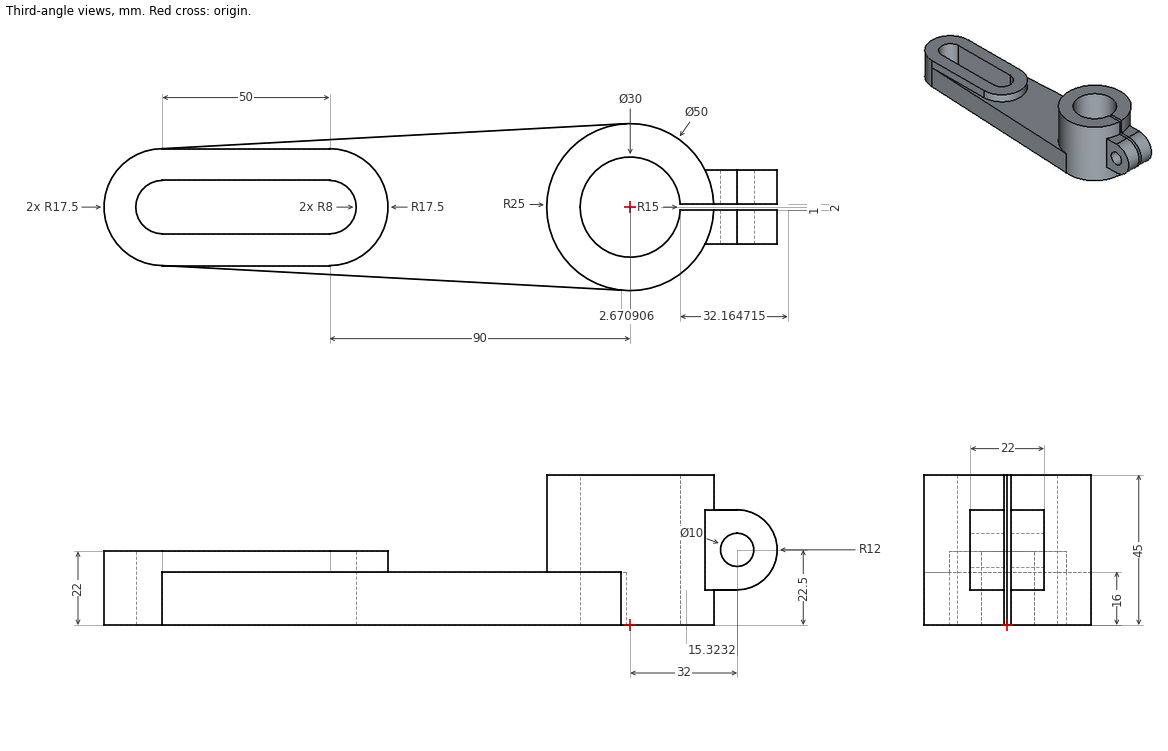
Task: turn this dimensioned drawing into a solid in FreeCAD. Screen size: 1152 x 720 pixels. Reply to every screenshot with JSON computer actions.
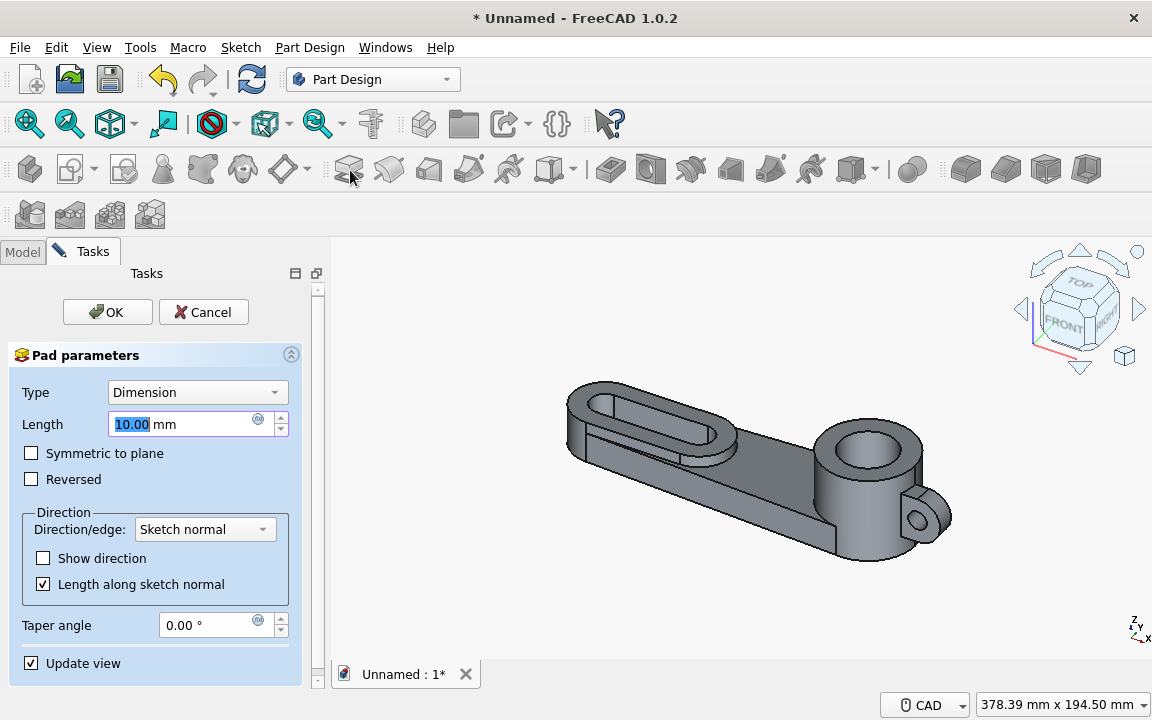
{"action": "type", "text": "22"}
{"action": "key", "text": "Tab"}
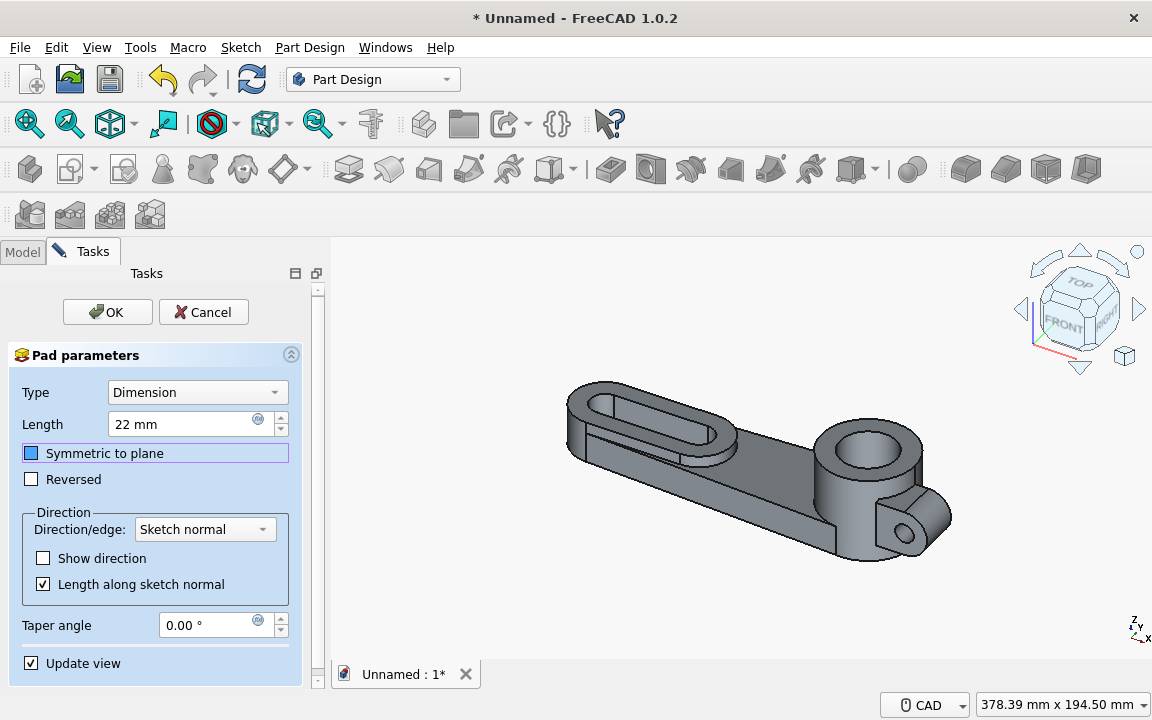
{"action": "left_click", "coordinate": [30, 453]}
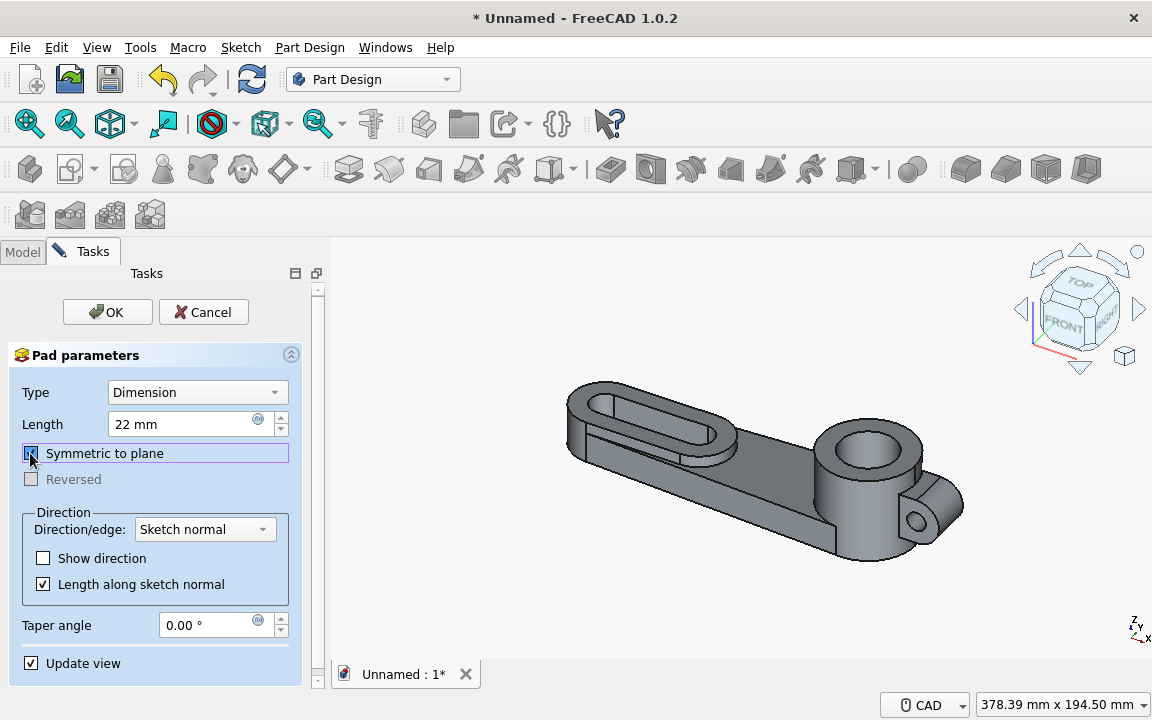
{"action": "left_click", "coordinate": [108, 312]}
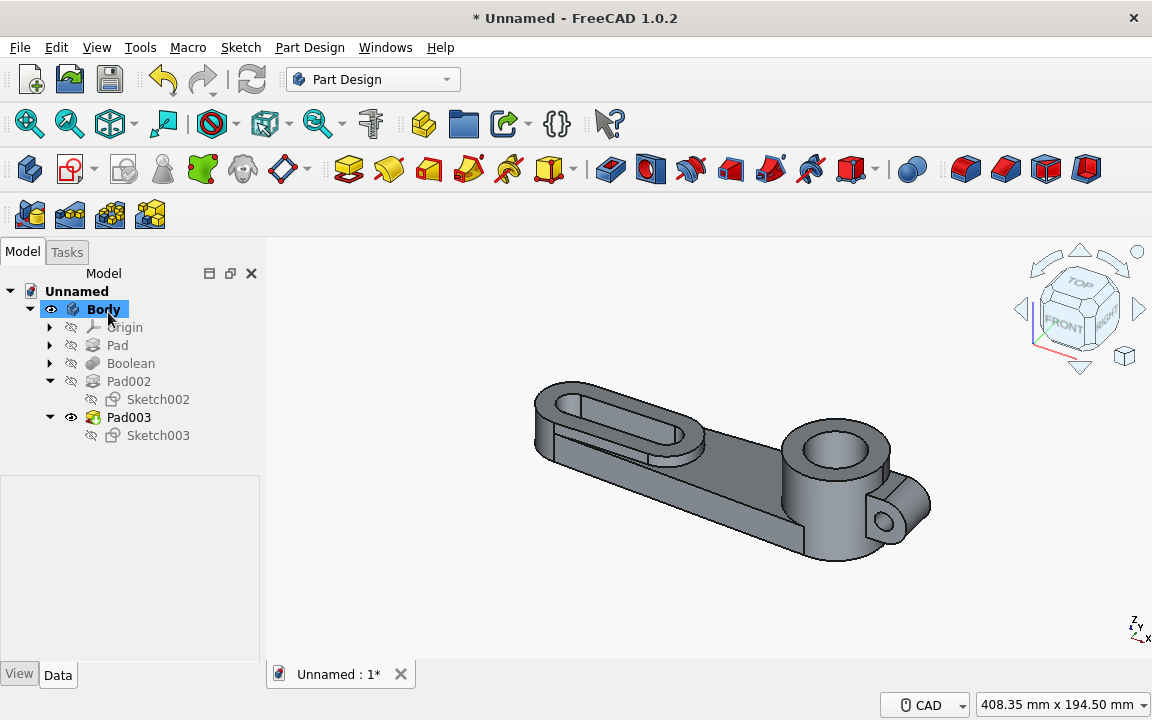
{"action": "left_click", "coordinate": [878, 443]}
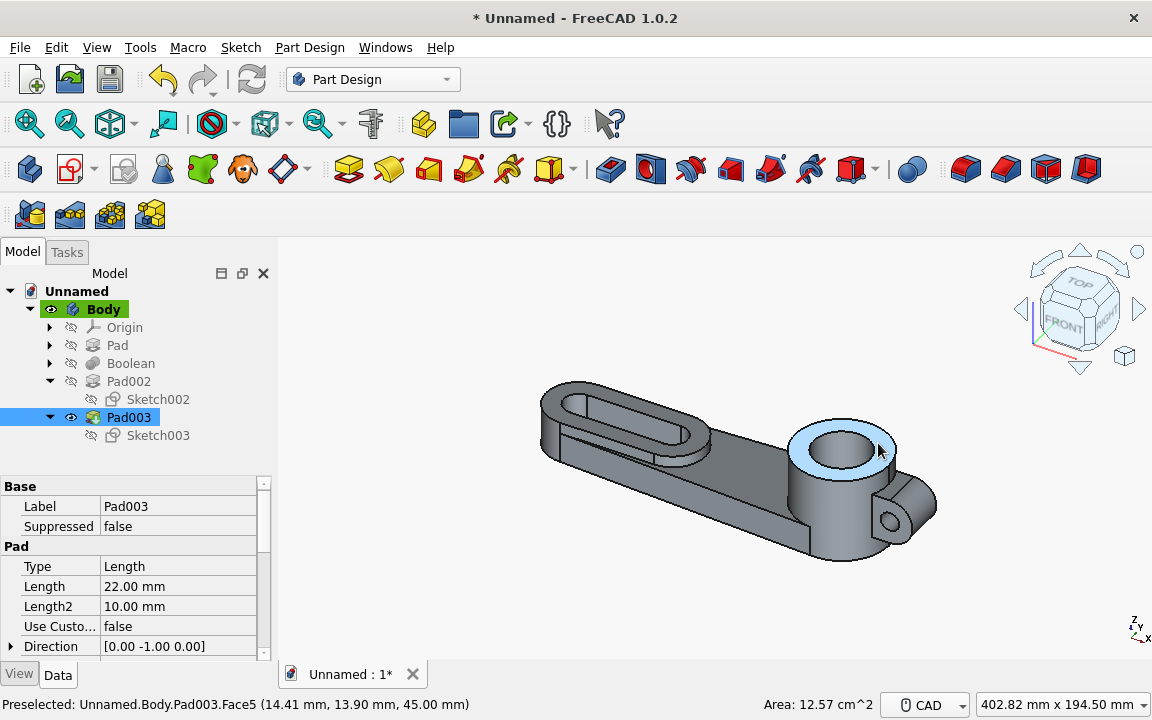
{"action": "left_click", "coordinate": [70, 170]}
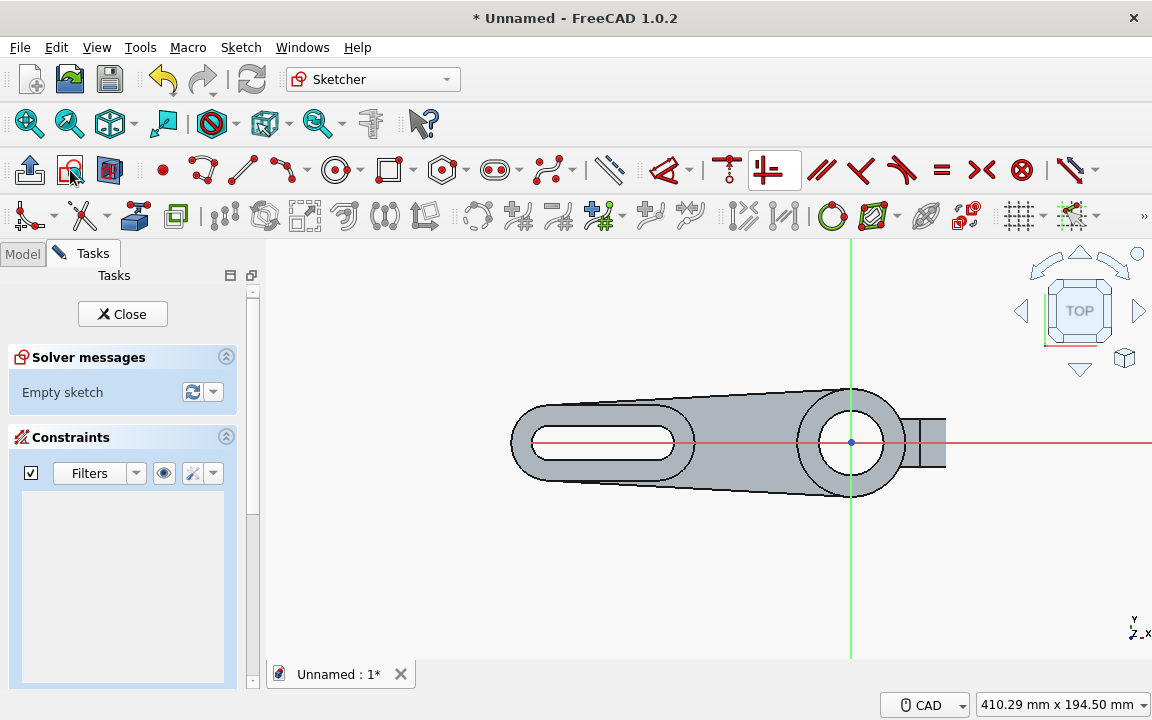
{"action": "scroll", "coordinate": [968, 441], "scroll_direction": "up", "scroll_amount": 8}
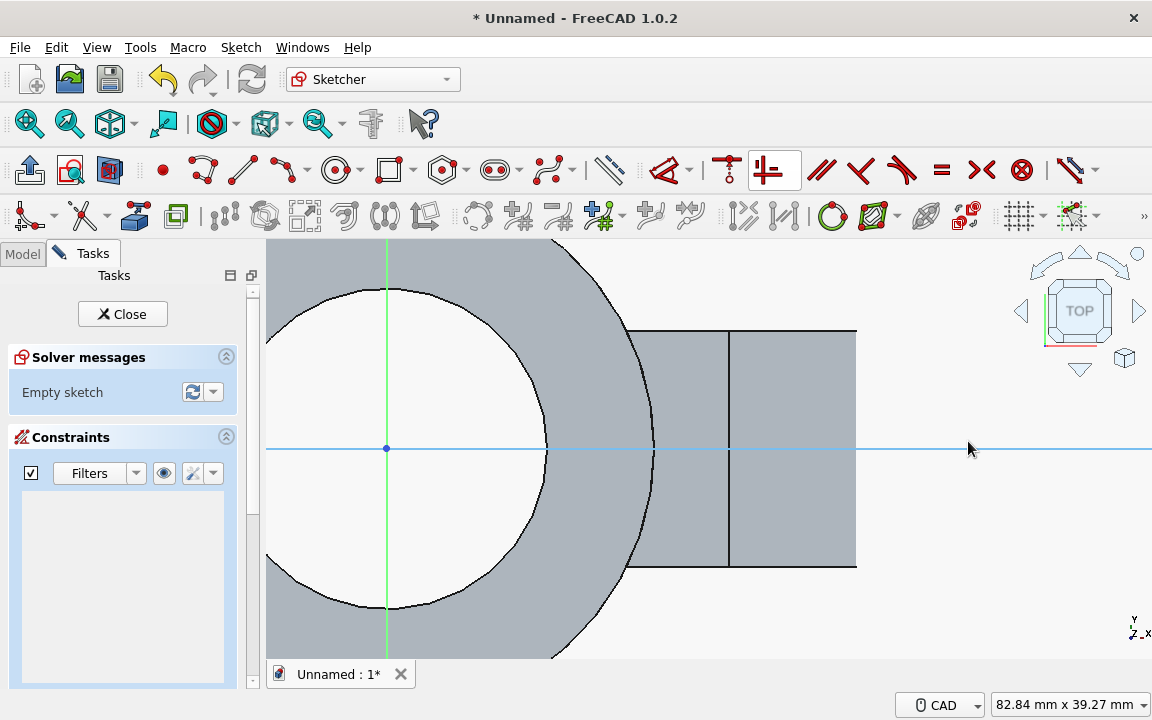
{"action": "key", "text": "g m"}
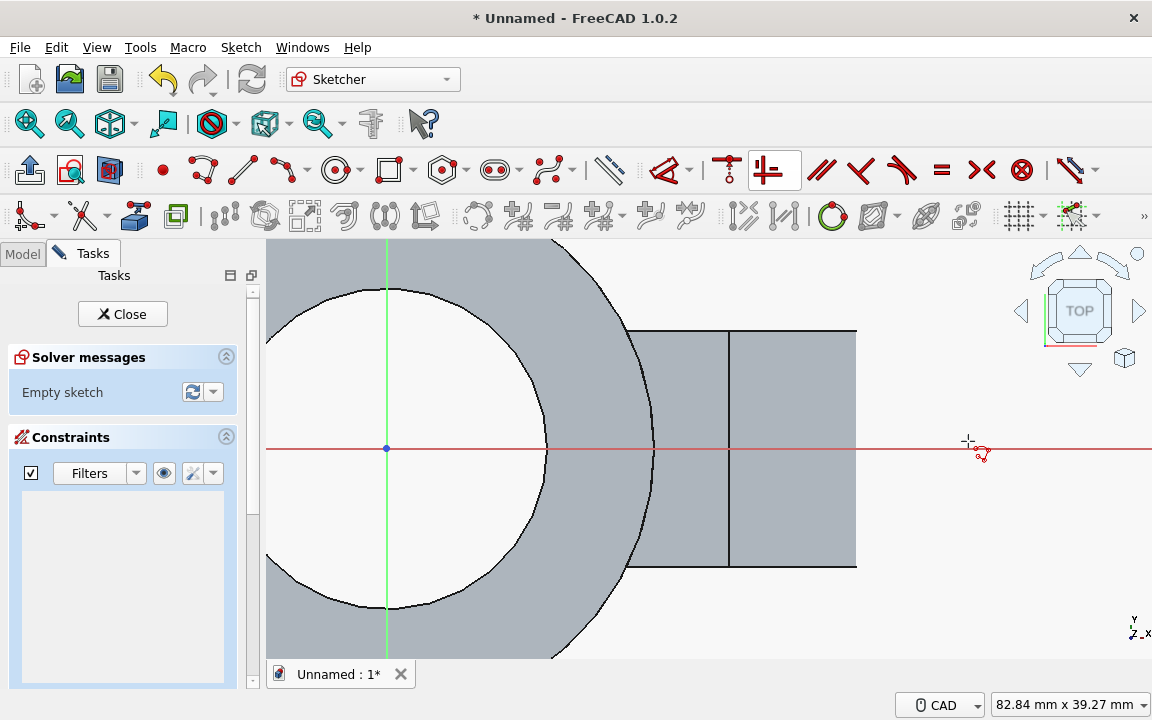
{"action": "scroll", "coordinate": [547, 460], "scroll_direction": "up", "scroll_amount": 2}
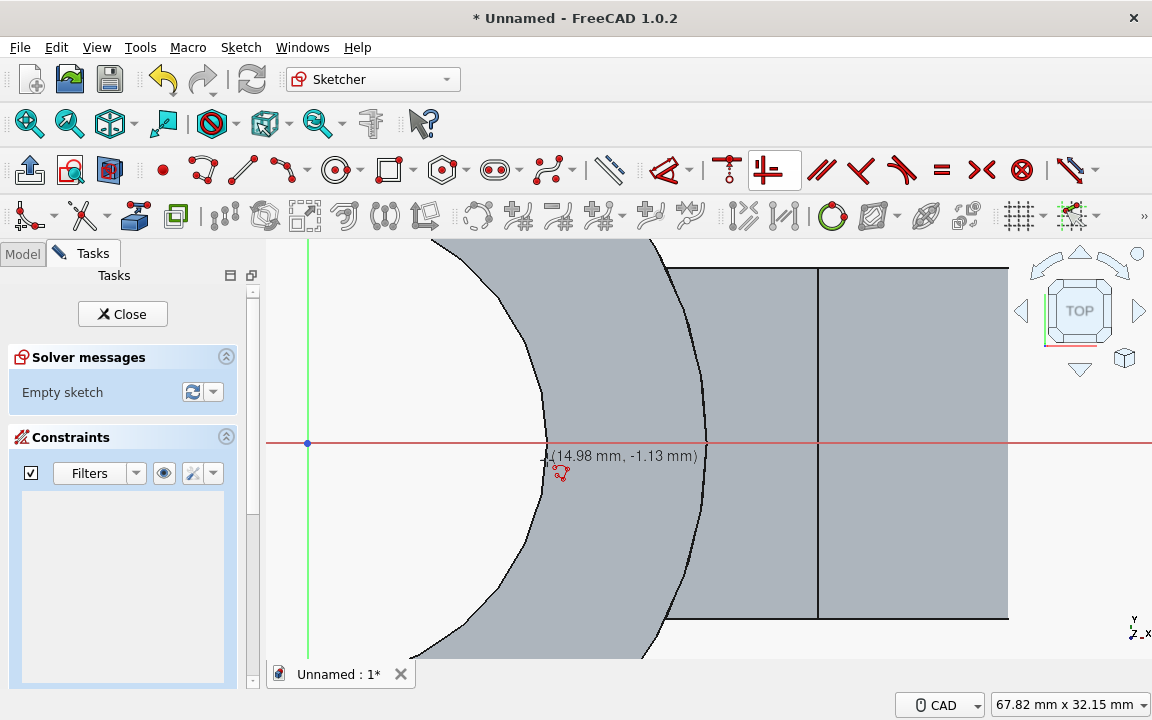
{"action": "left_click", "coordinate": [547, 459]}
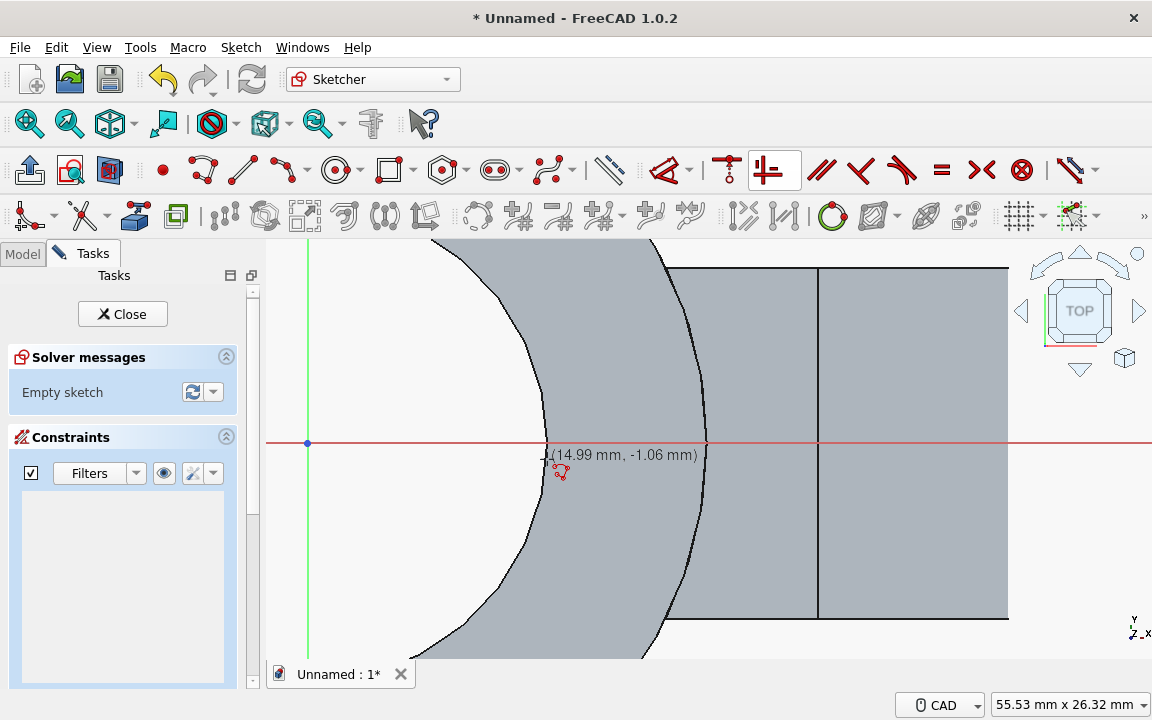
{"action": "scroll", "coordinate": [552, 461], "scroll_direction": "down", "scroll_amount": 2}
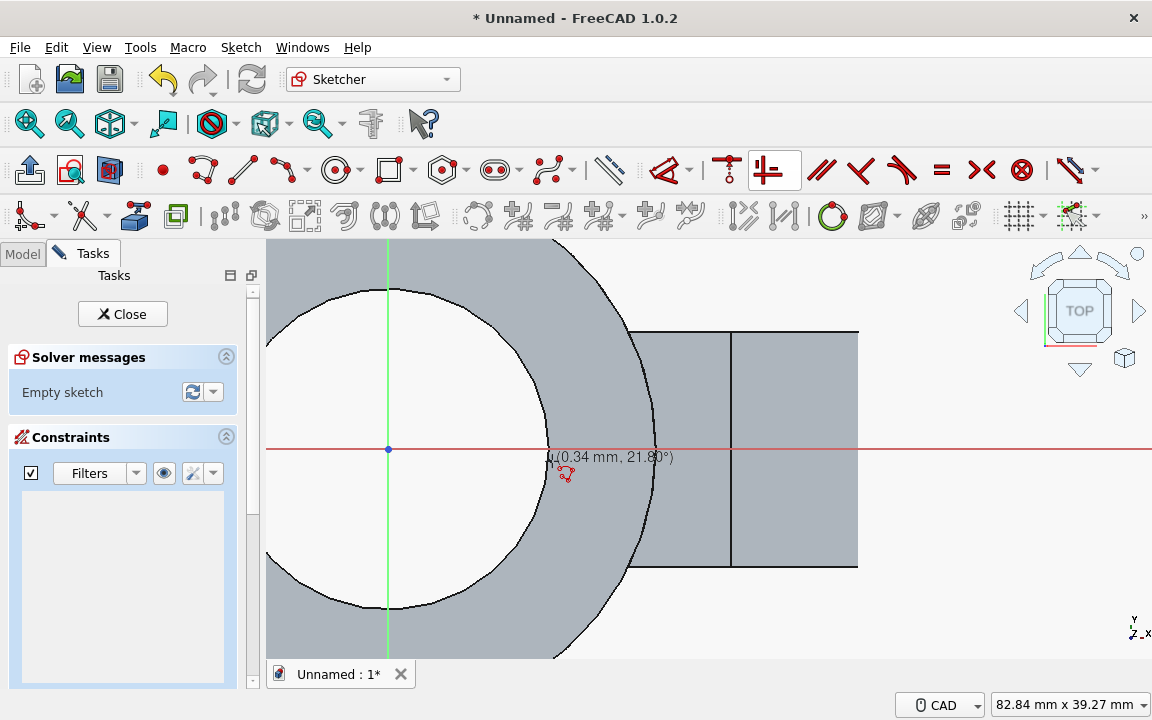
{"action": "scroll", "coordinate": [893, 460], "scroll_direction": "up", "scroll_amount": 2}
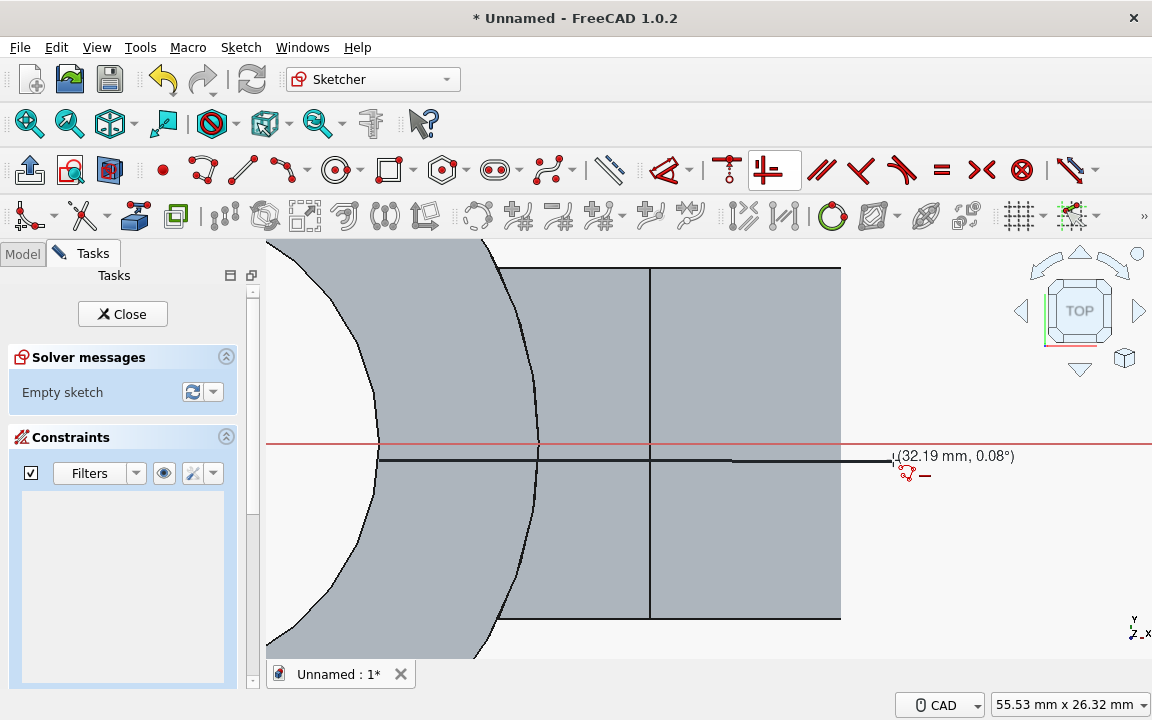
{"action": "left_click", "coordinate": [892, 459]}
{"action": "left_click", "coordinate": [892, 428]}
{"action": "left_click", "coordinate": [379, 428]}
{"action": "right_click", "coordinate": [379, 428]}